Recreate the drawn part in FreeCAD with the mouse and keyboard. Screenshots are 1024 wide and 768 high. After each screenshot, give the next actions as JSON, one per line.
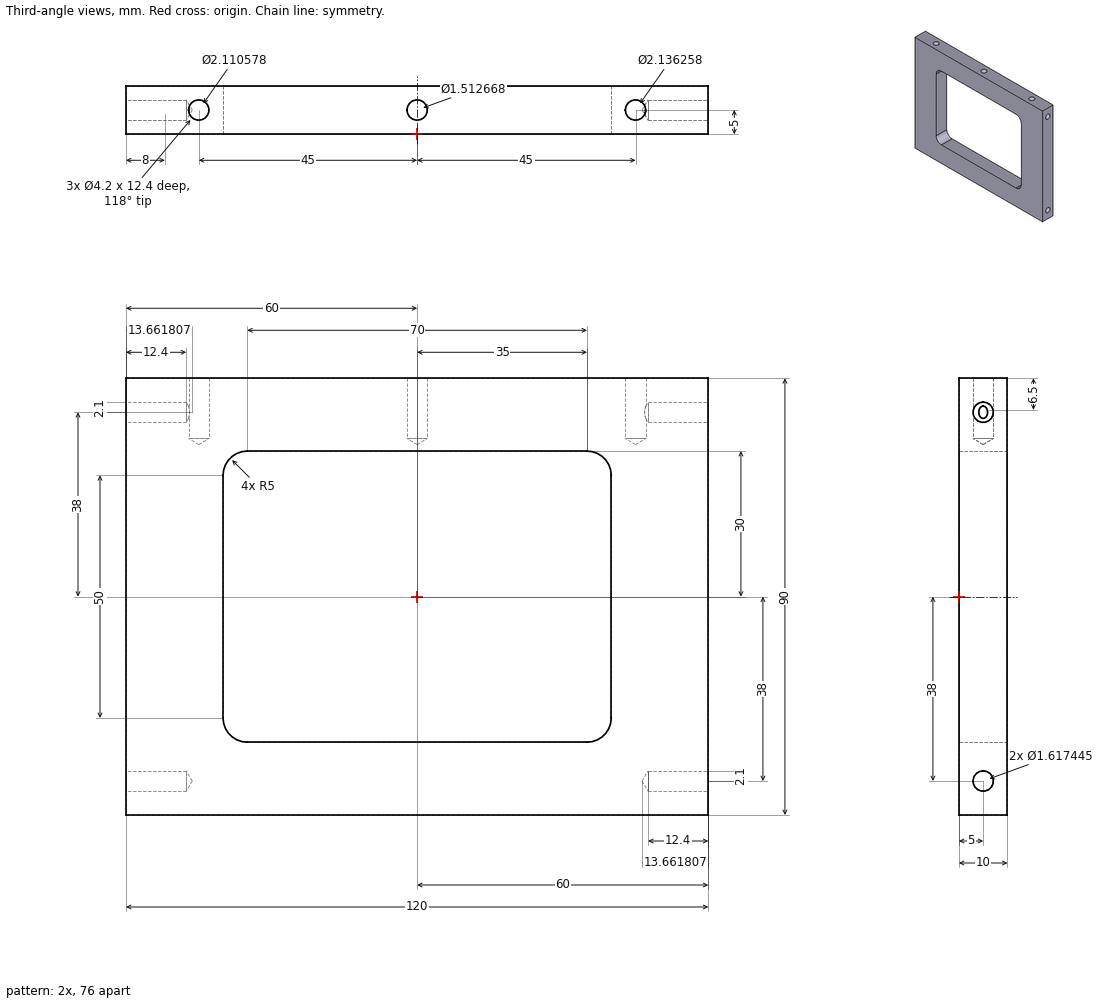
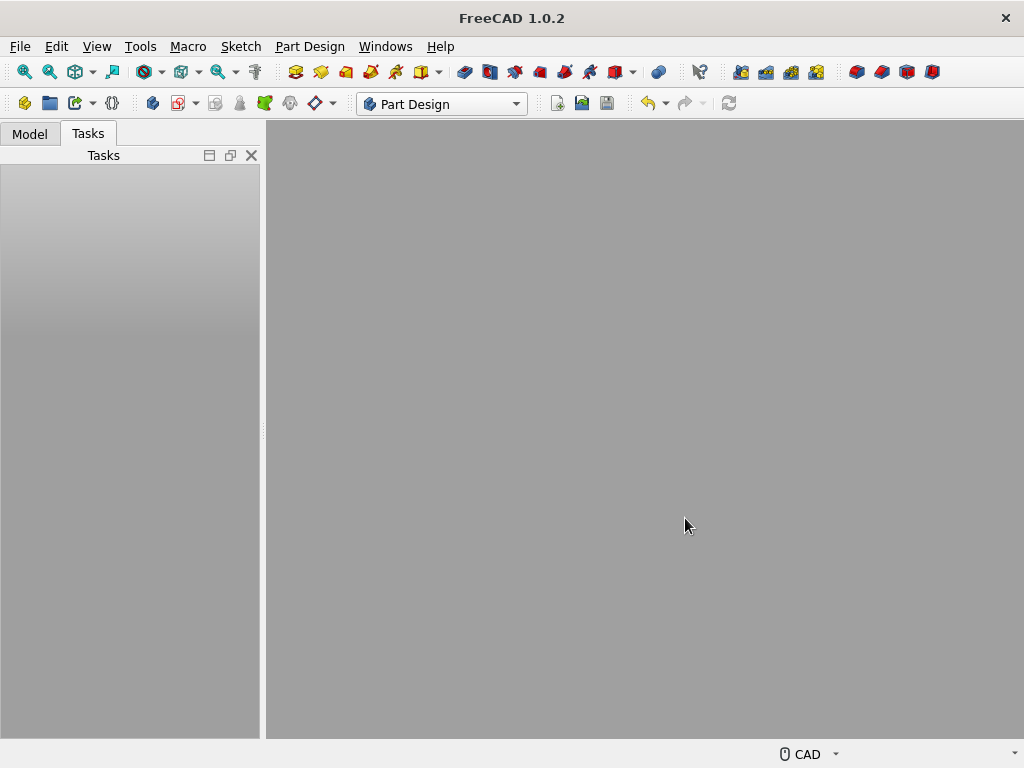
{"action": "left_click", "coordinate": [557, 104]}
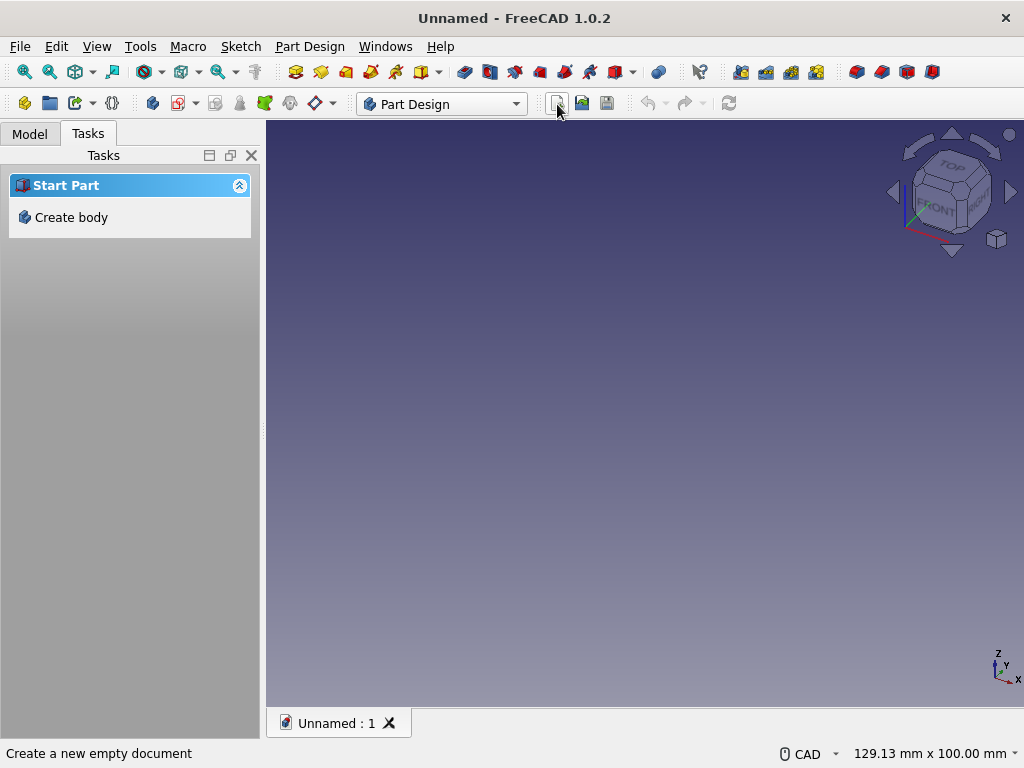
{"action": "left_click", "coordinate": [178, 104]}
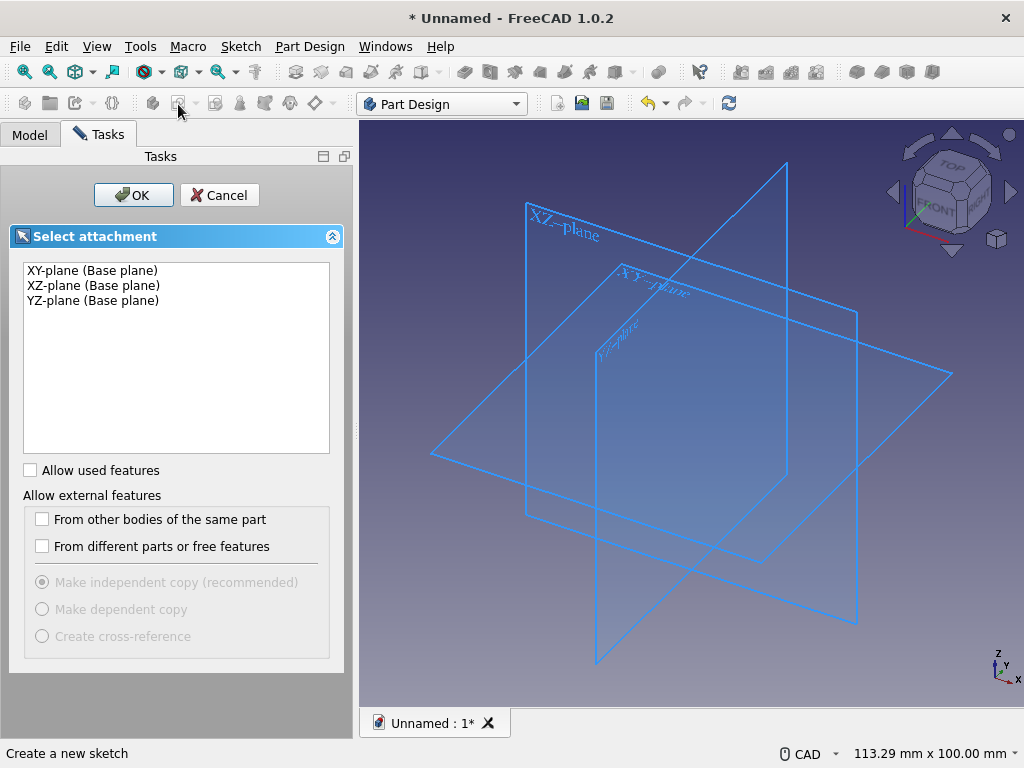
{"action": "left_click", "coordinate": [84, 286]}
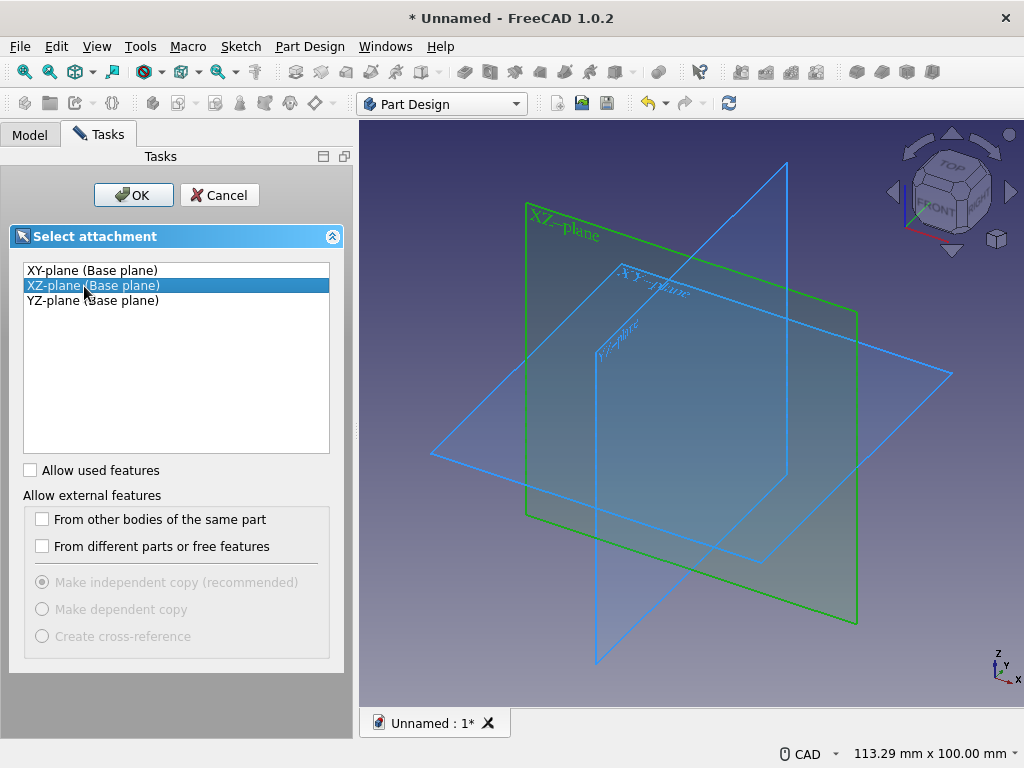
{"action": "left_click", "coordinate": [134, 195]}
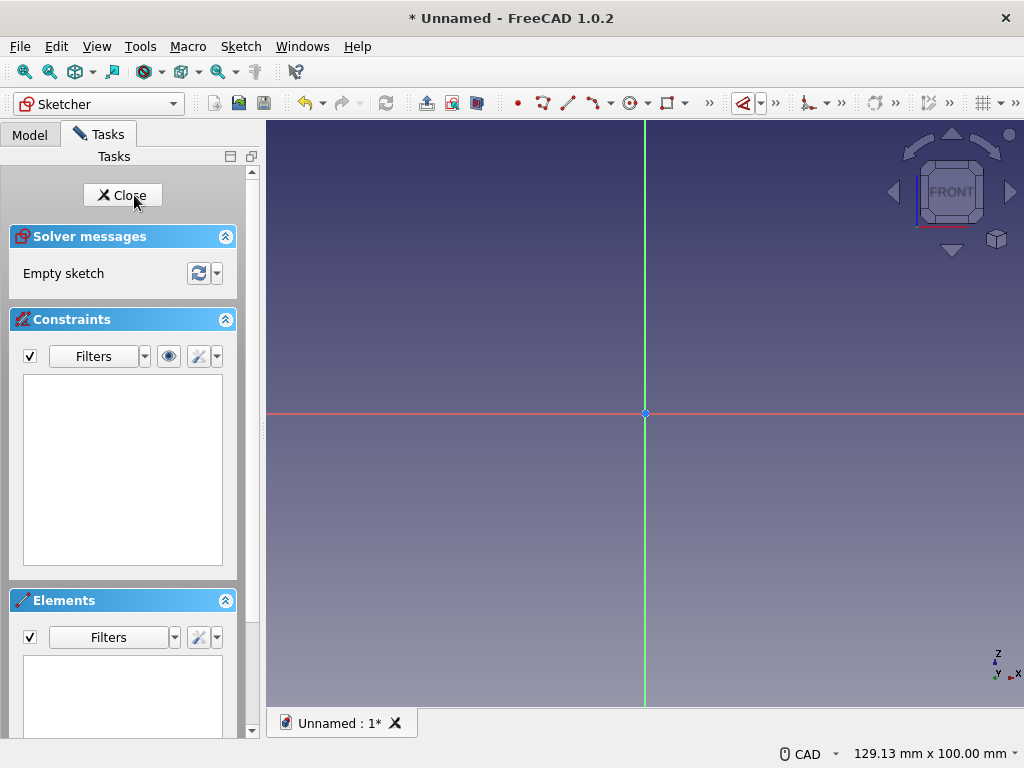
{"action": "scroll", "coordinate": [493, 414], "scroll_direction": "down", "scroll_amount": 3}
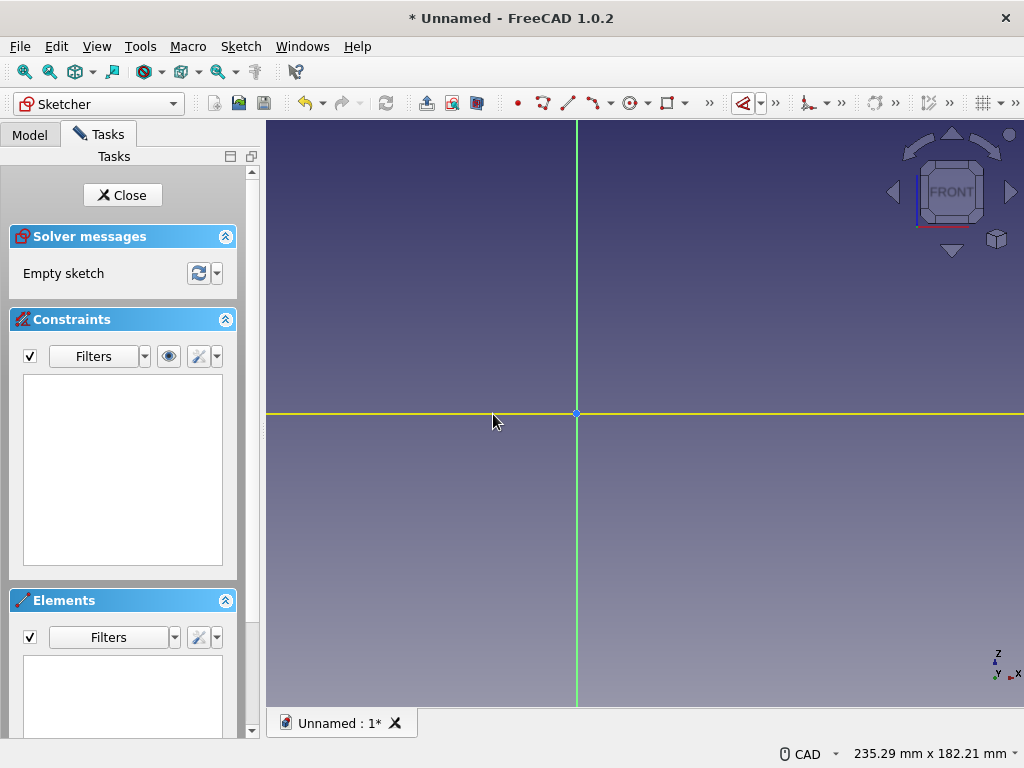
{"action": "left_click", "coordinate": [684, 104]}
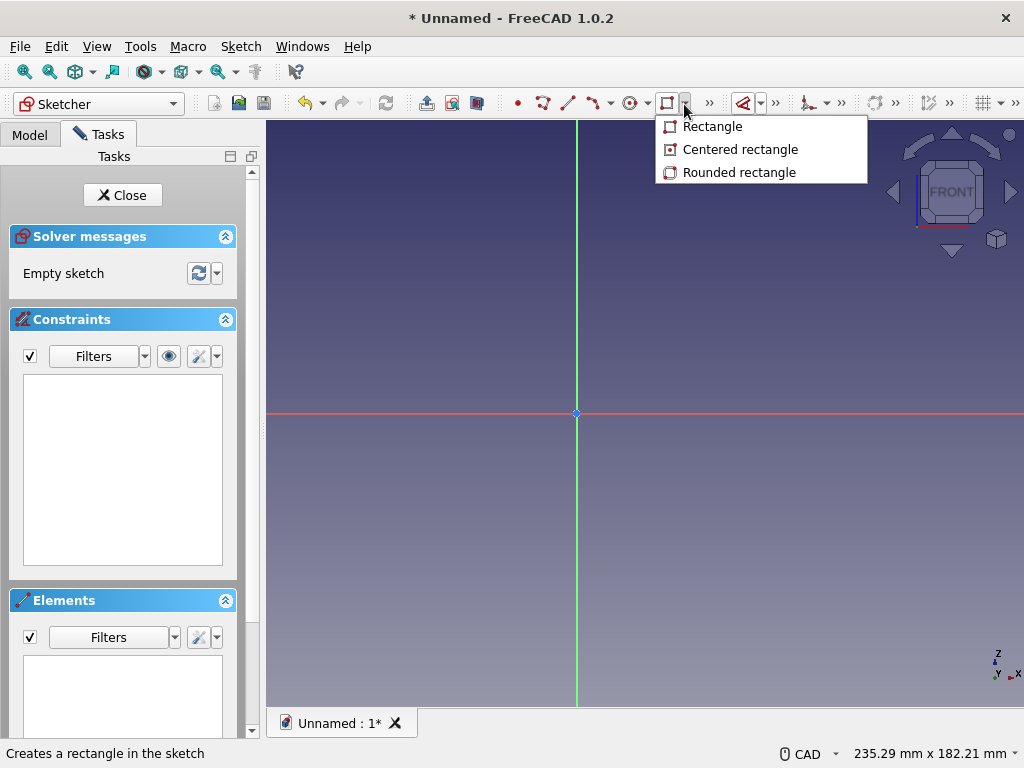
{"action": "left_click", "coordinate": [762, 150]}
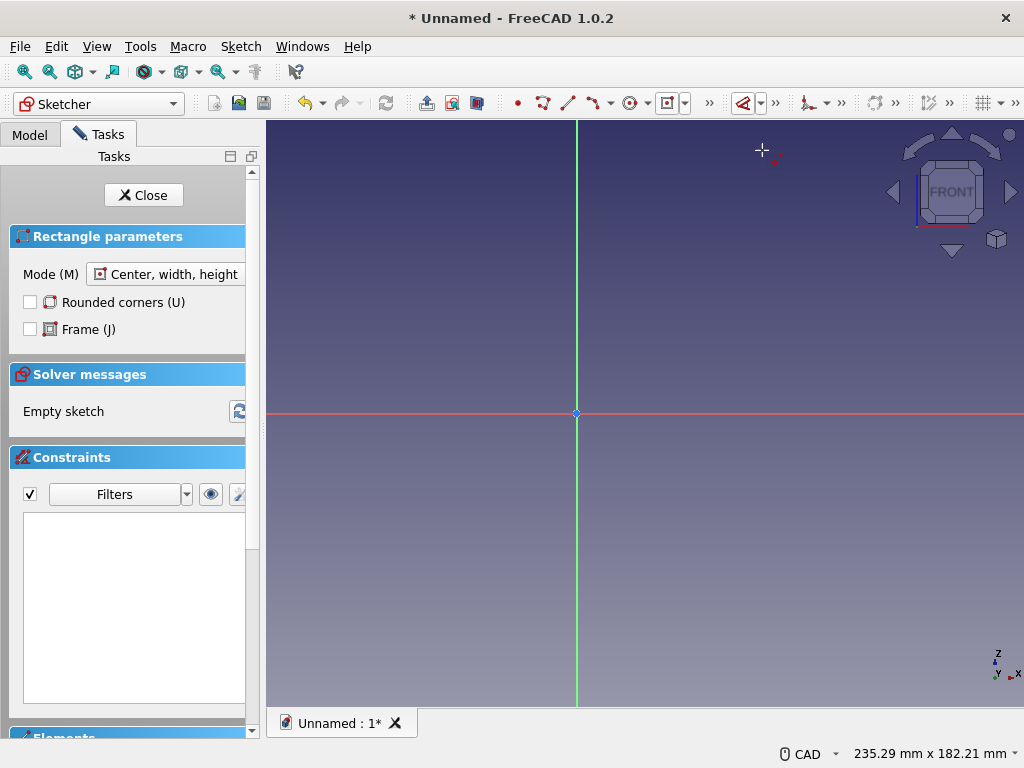
{"action": "left_click", "coordinate": [577, 414]}
{"action": "mouse_move", "coordinate": [770, 269]}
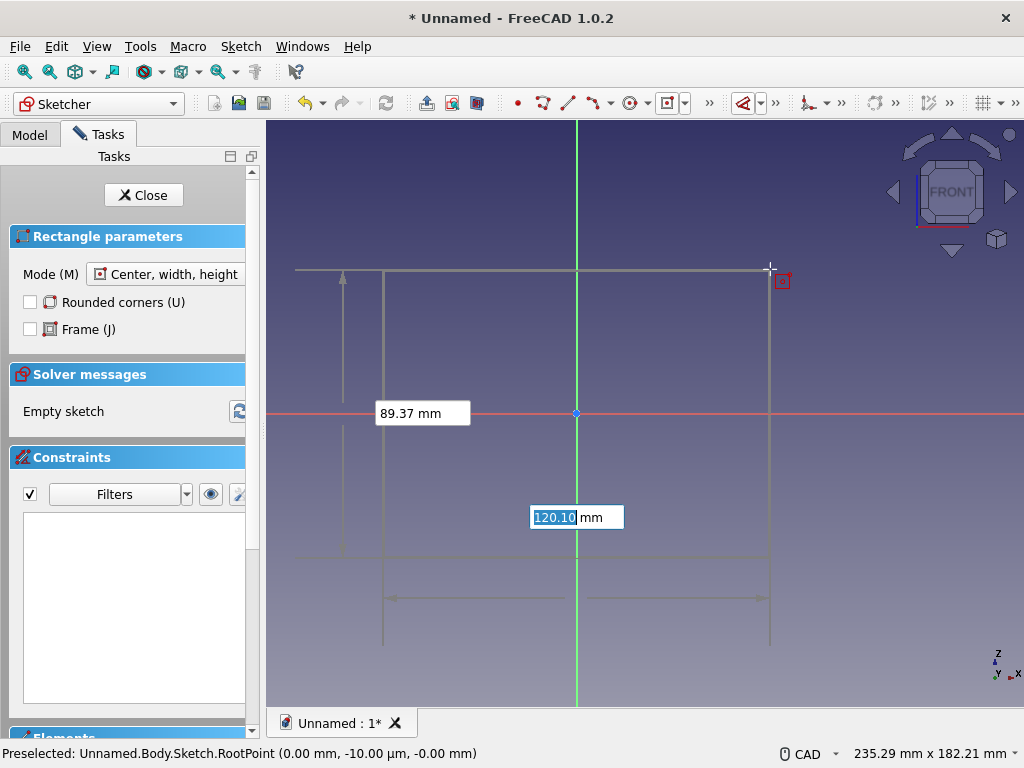
{"action": "type", "text": "120"}
{"action": "key", "text": "Tab"}
{"action": "type", "text": "90"}
{"action": "key", "text": "Return"}
{"action": "key", "text": "Escape"}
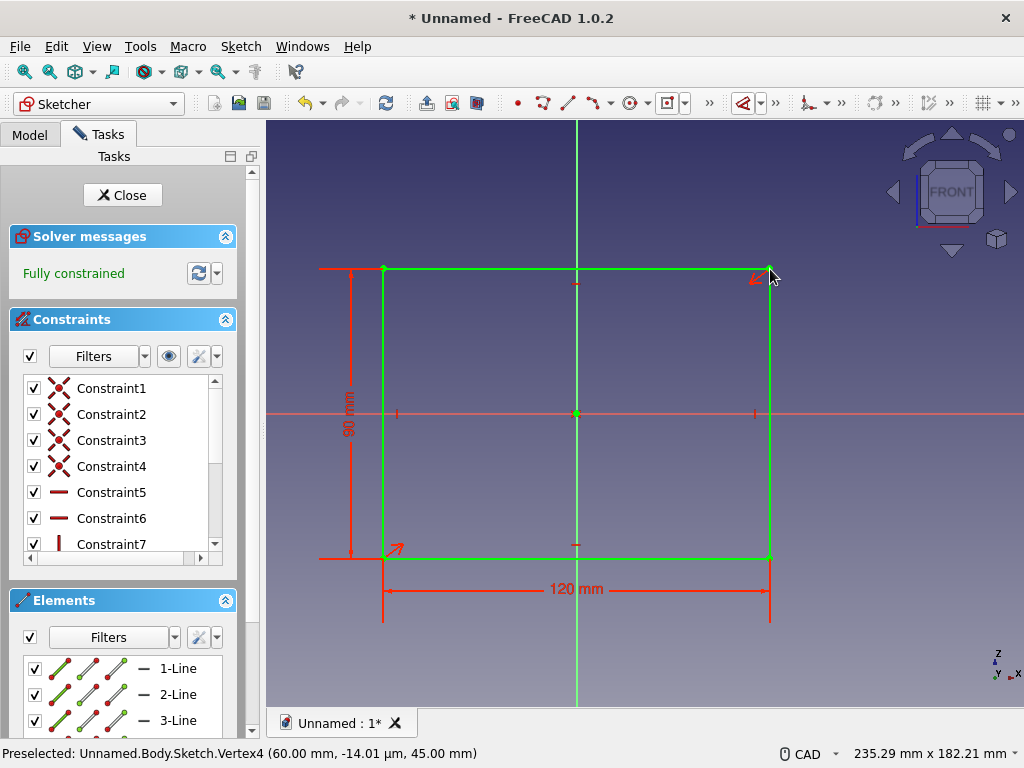
{"action": "left_click", "coordinate": [123, 195]}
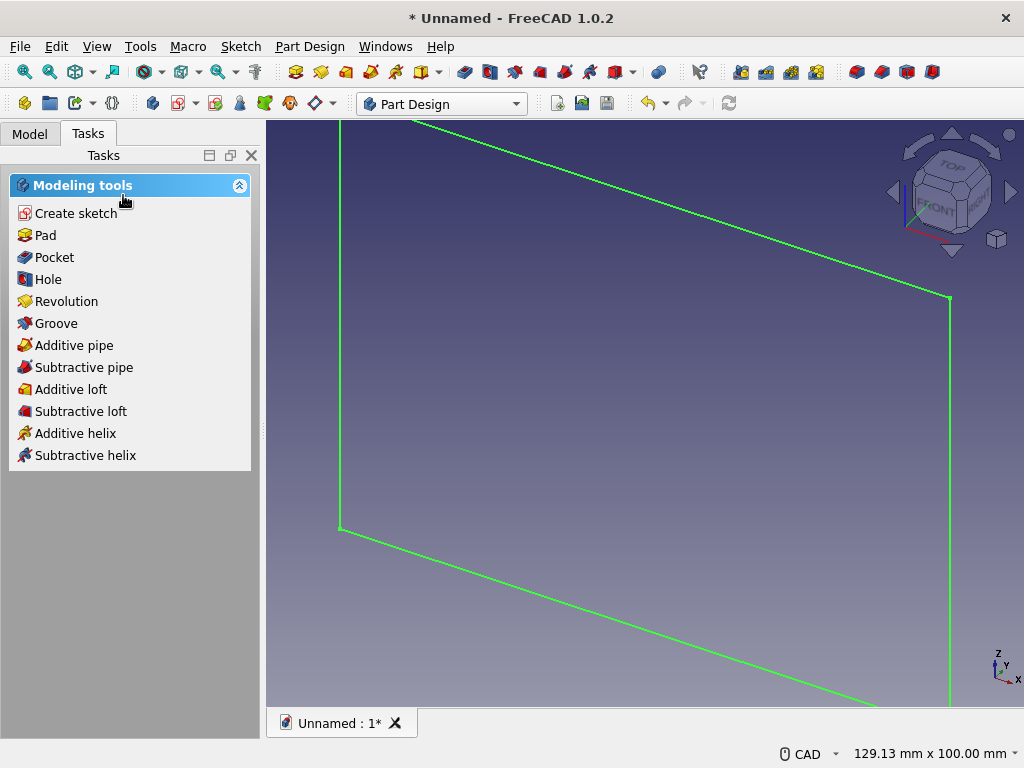
{"action": "left_click", "coordinate": [296, 72]}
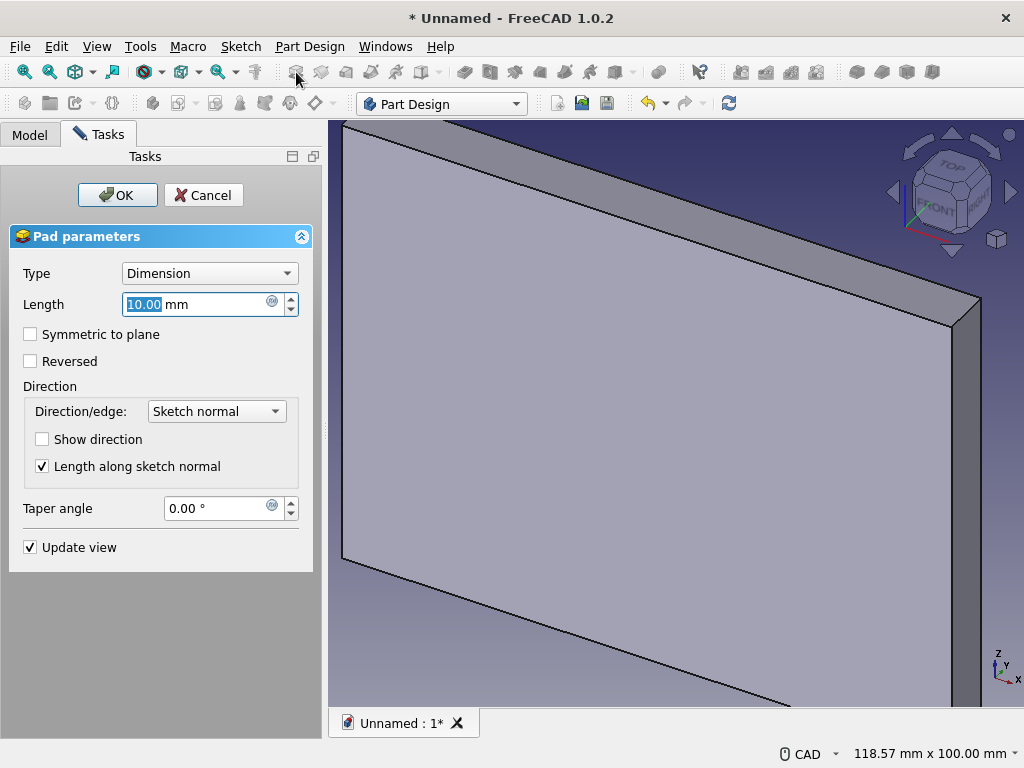
{"action": "type", "text": "10"}
{"action": "key", "text": "Tab"}